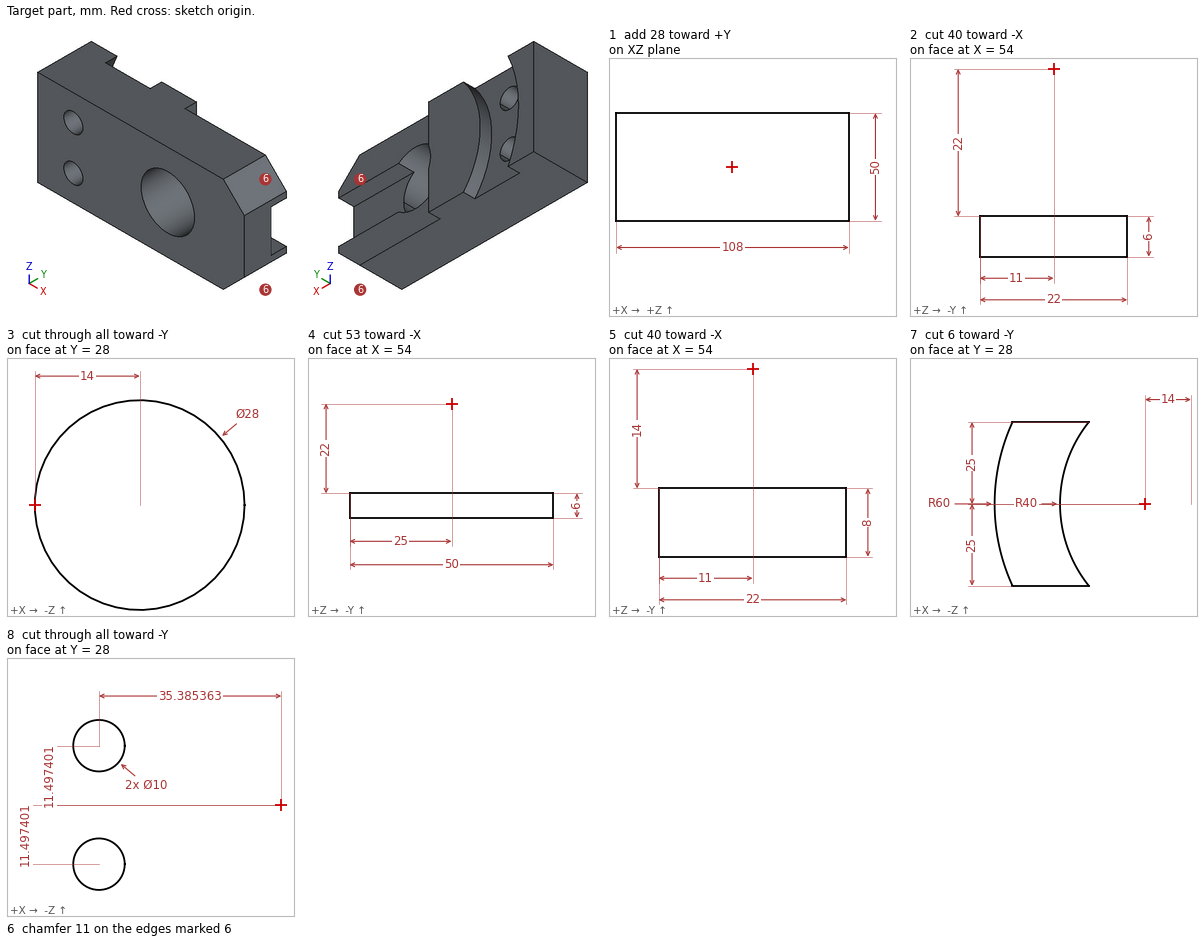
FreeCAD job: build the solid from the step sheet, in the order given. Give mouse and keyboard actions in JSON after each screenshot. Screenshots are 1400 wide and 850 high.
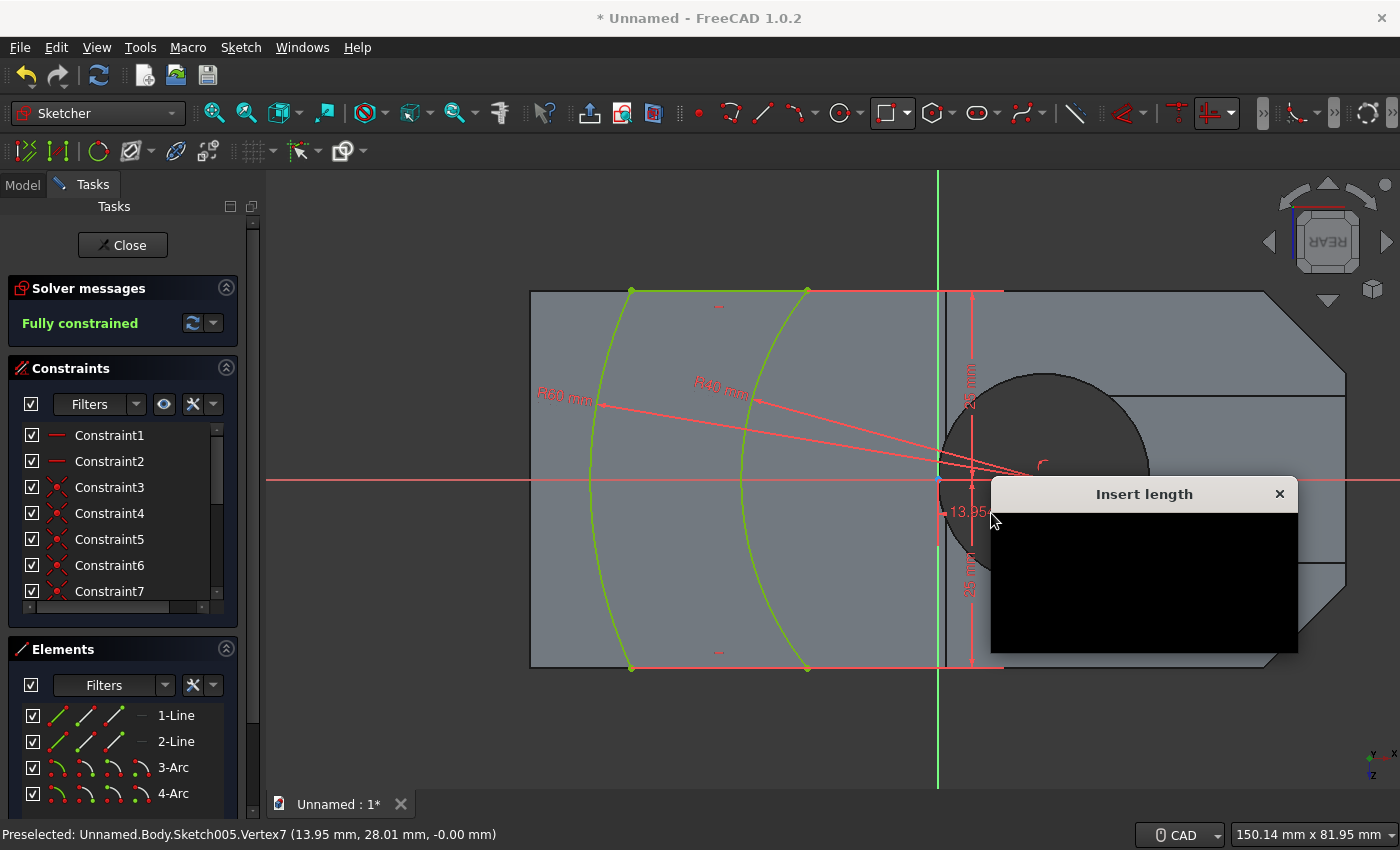
{"action": "type", "text": "14"}
{"action": "key", "text": "Return"}
{"action": "key", "text": "Escape"}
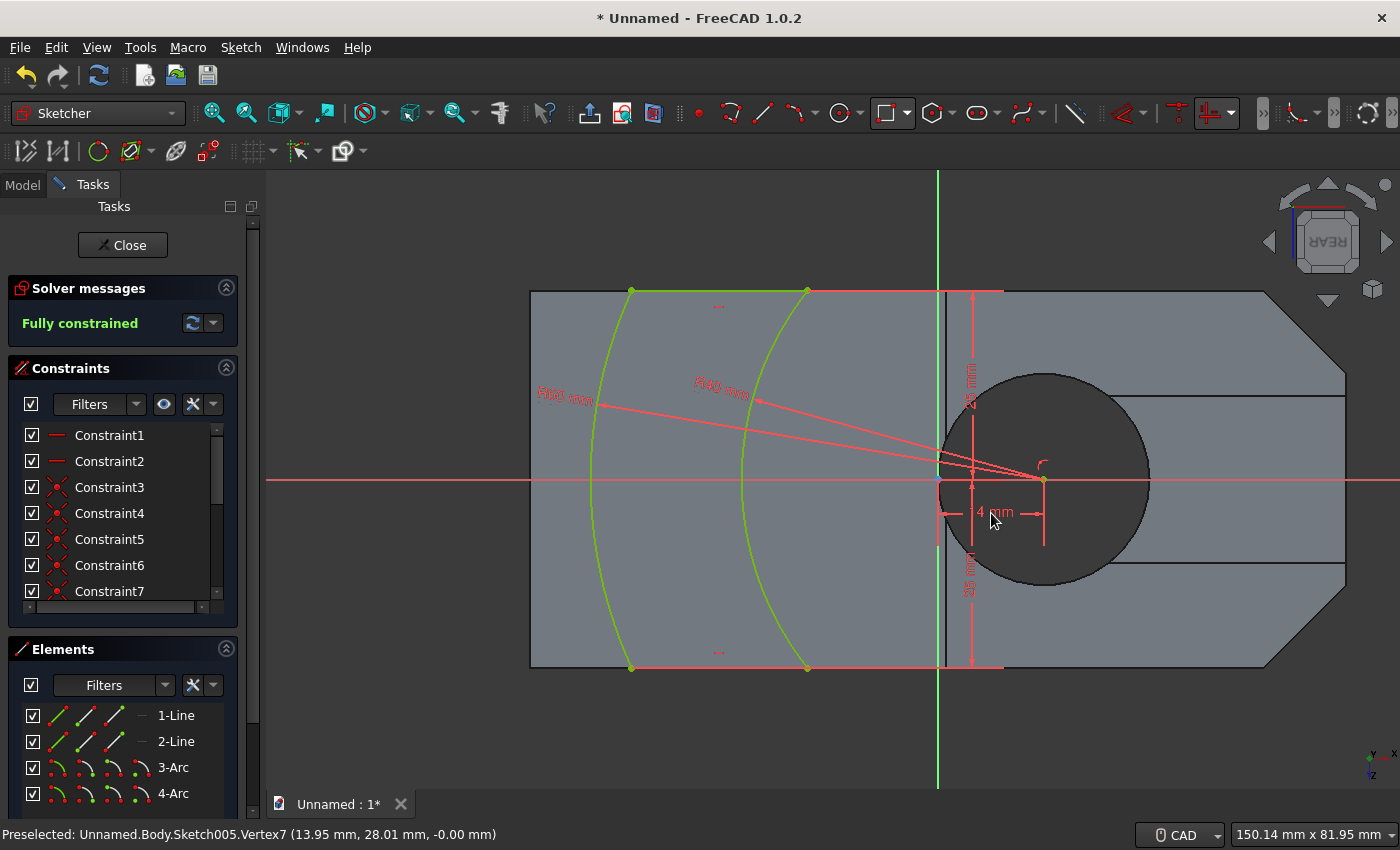
{"action": "left_click", "coordinate": [123, 245]}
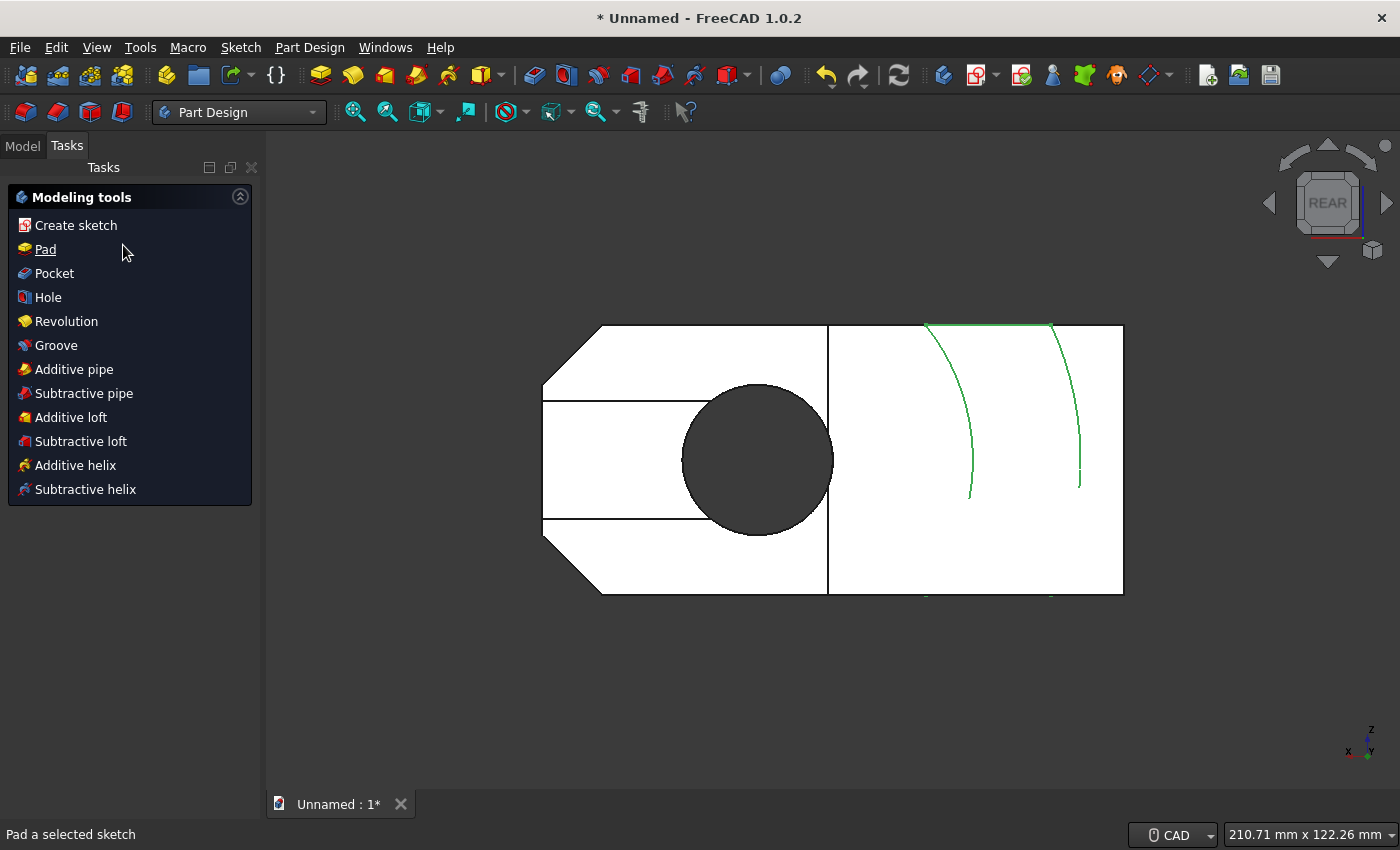
{"action": "left_click", "coordinate": [536, 76]}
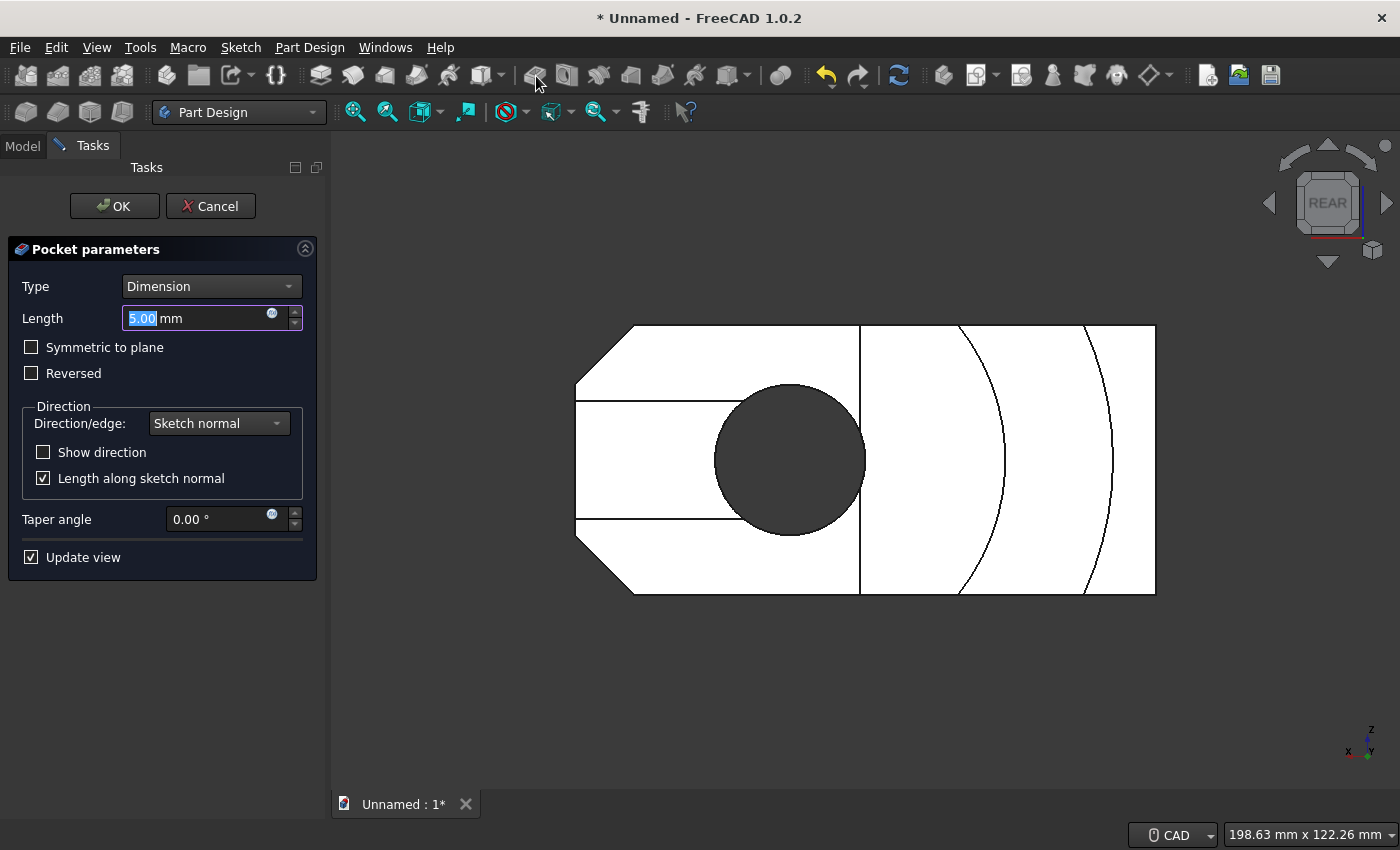
{"action": "type", "text": "6"}
{"action": "key", "text": "Tab"}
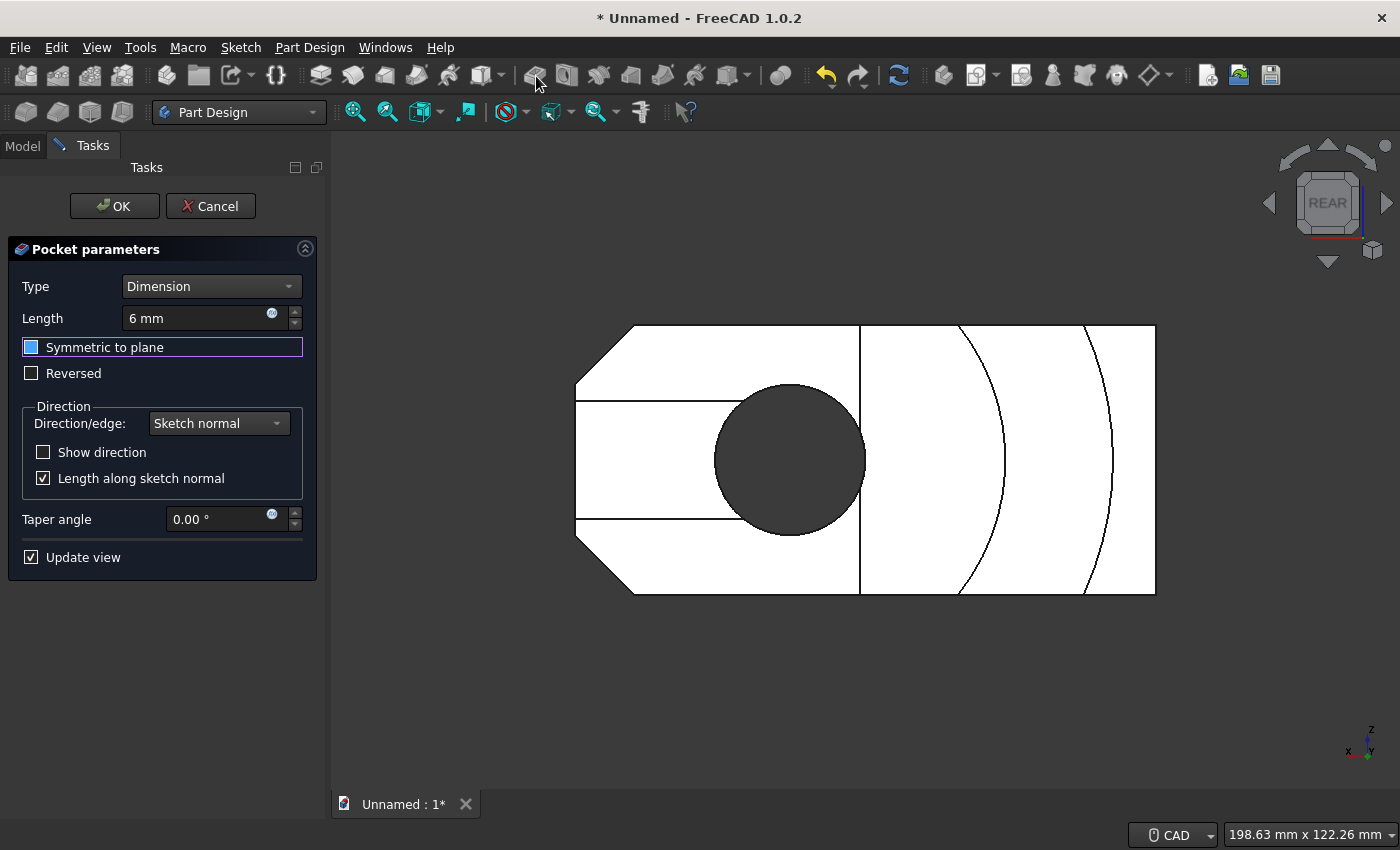
{"action": "left_click", "coordinate": [115, 206]}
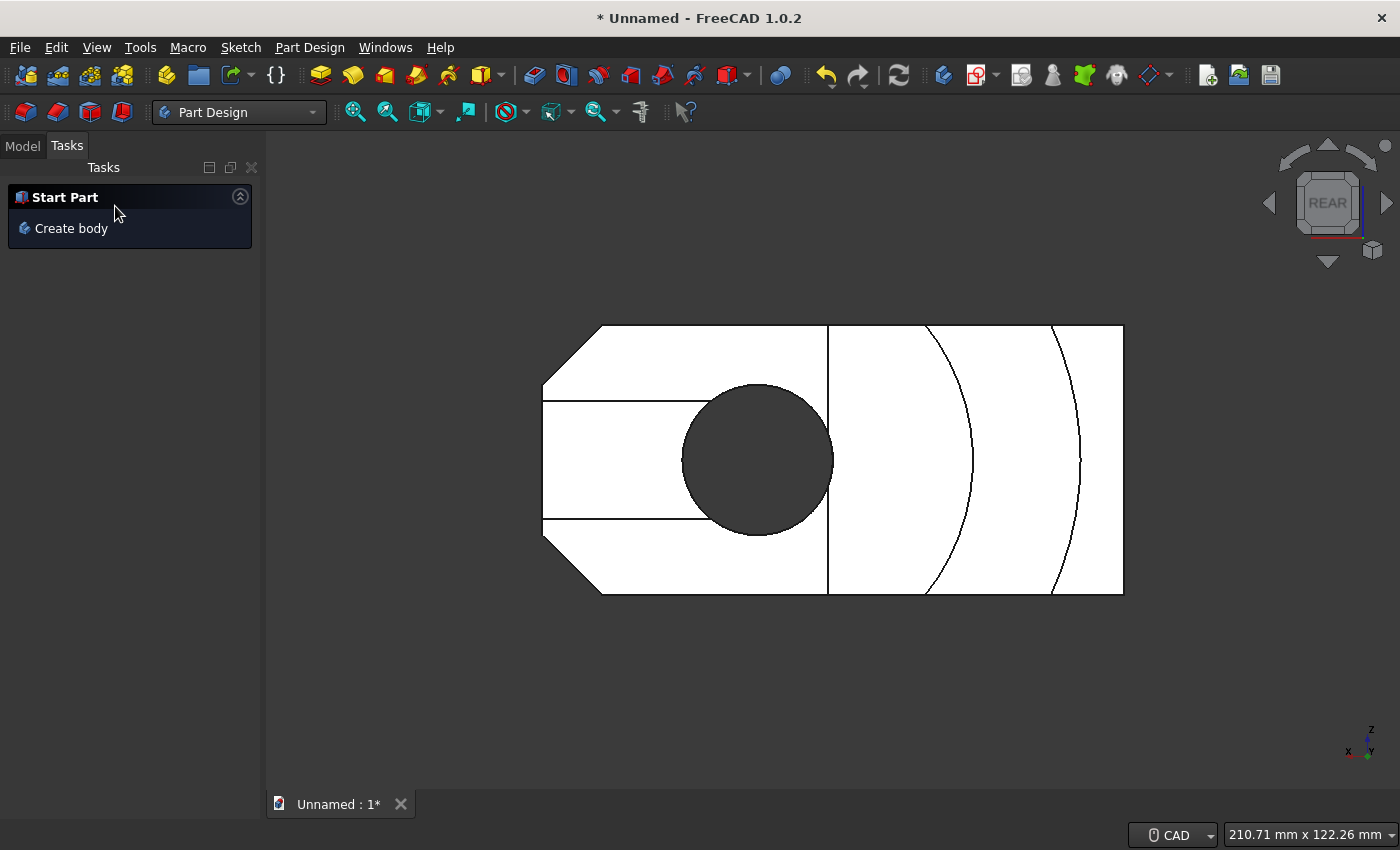
{"action": "left_click", "coordinate": [900, 497]}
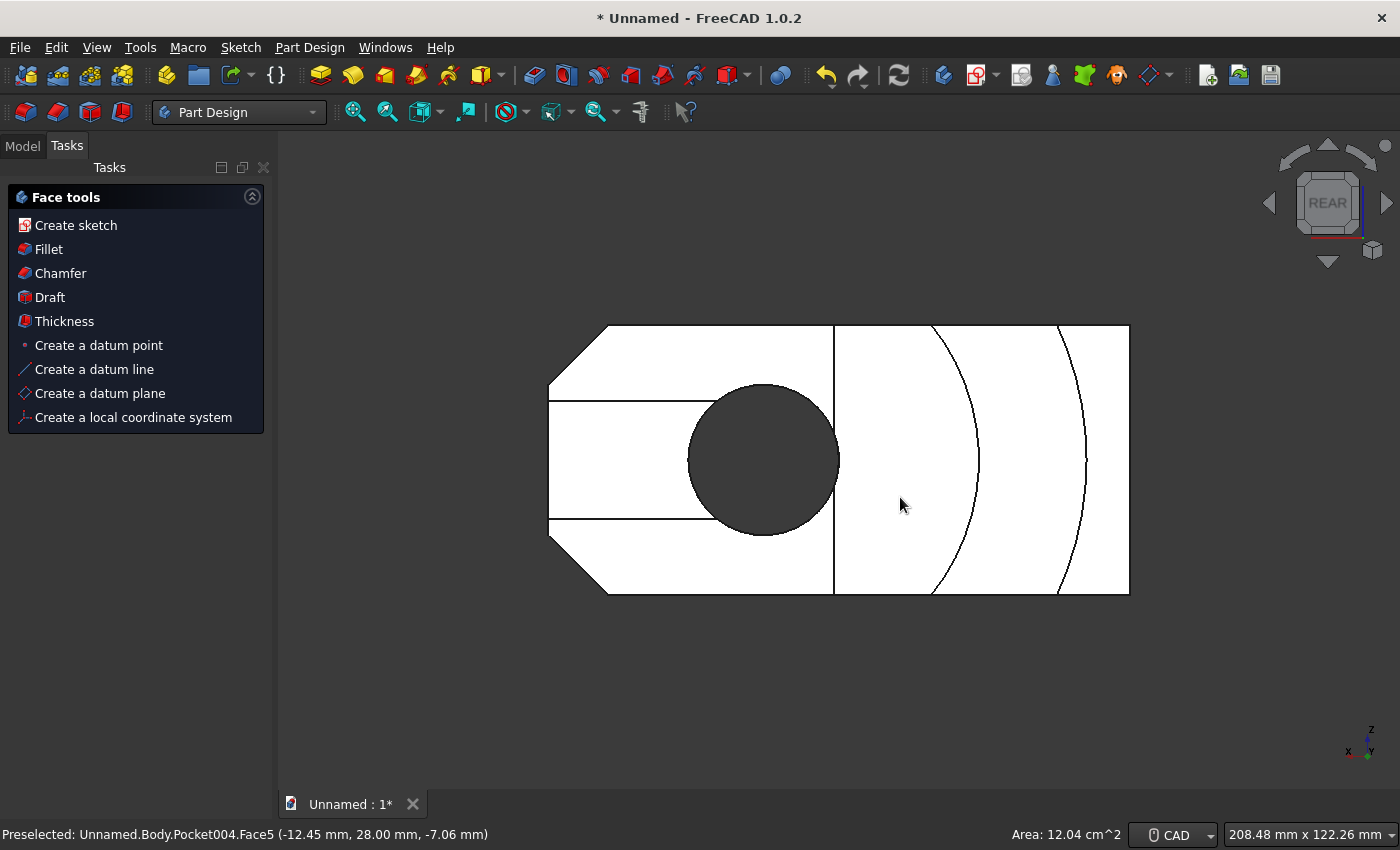
{"action": "left_click", "coordinate": [976, 76]}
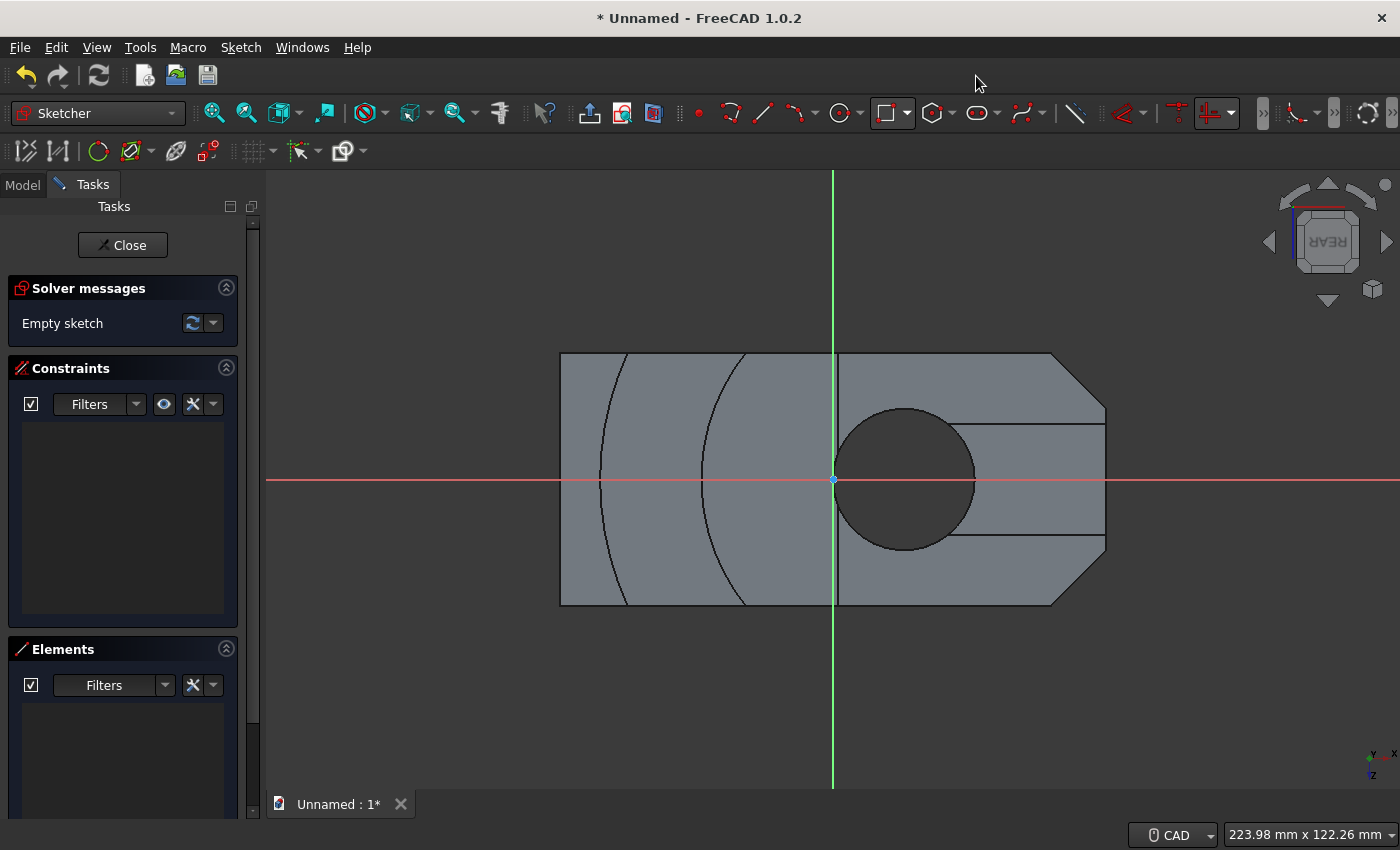
{"action": "scroll", "coordinate": [703, 479], "scroll_direction": "up", "scroll_amount": 4}